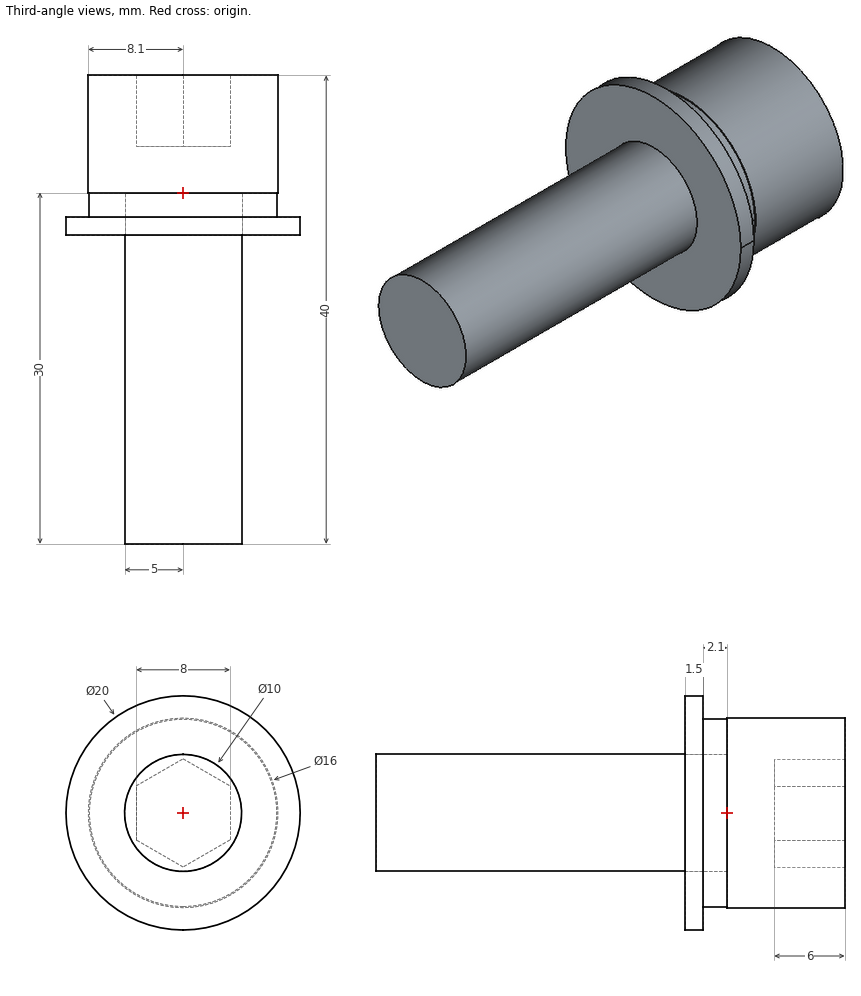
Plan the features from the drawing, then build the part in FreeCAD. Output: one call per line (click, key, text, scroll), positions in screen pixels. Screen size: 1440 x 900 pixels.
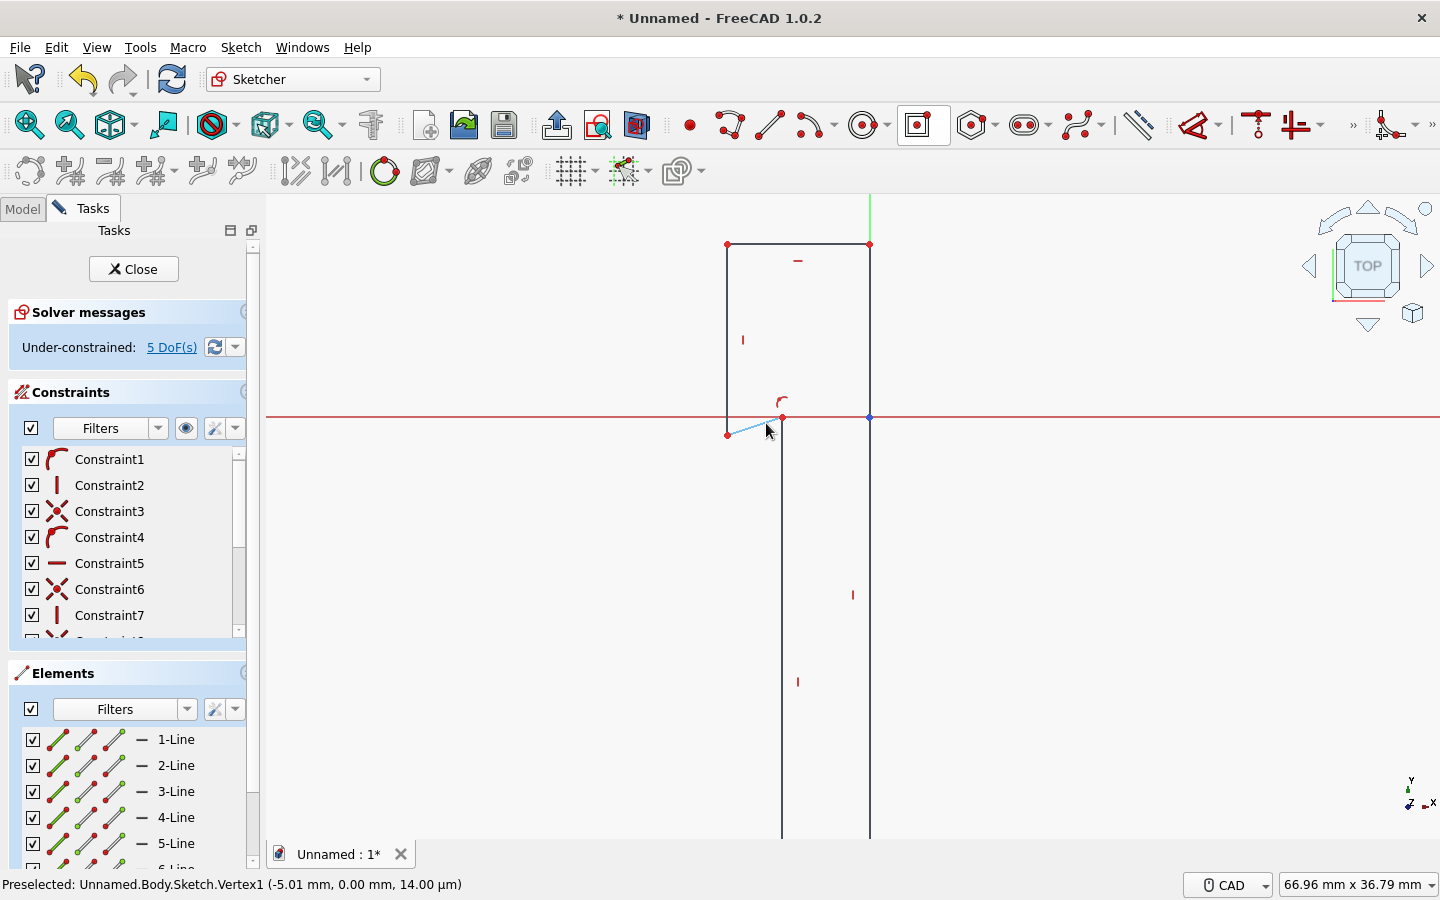
click(766, 423)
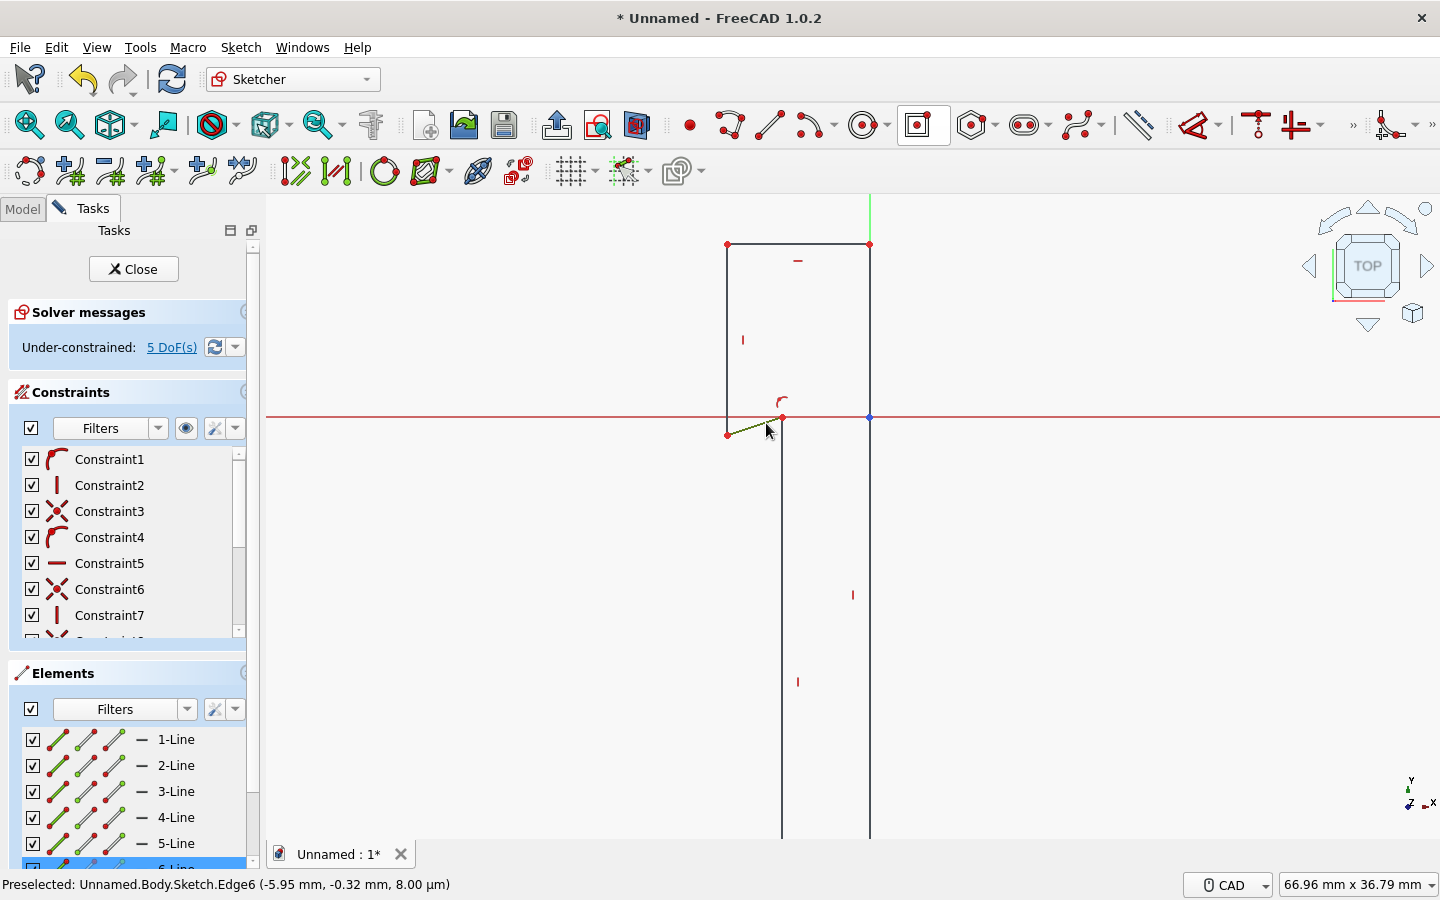
key(h)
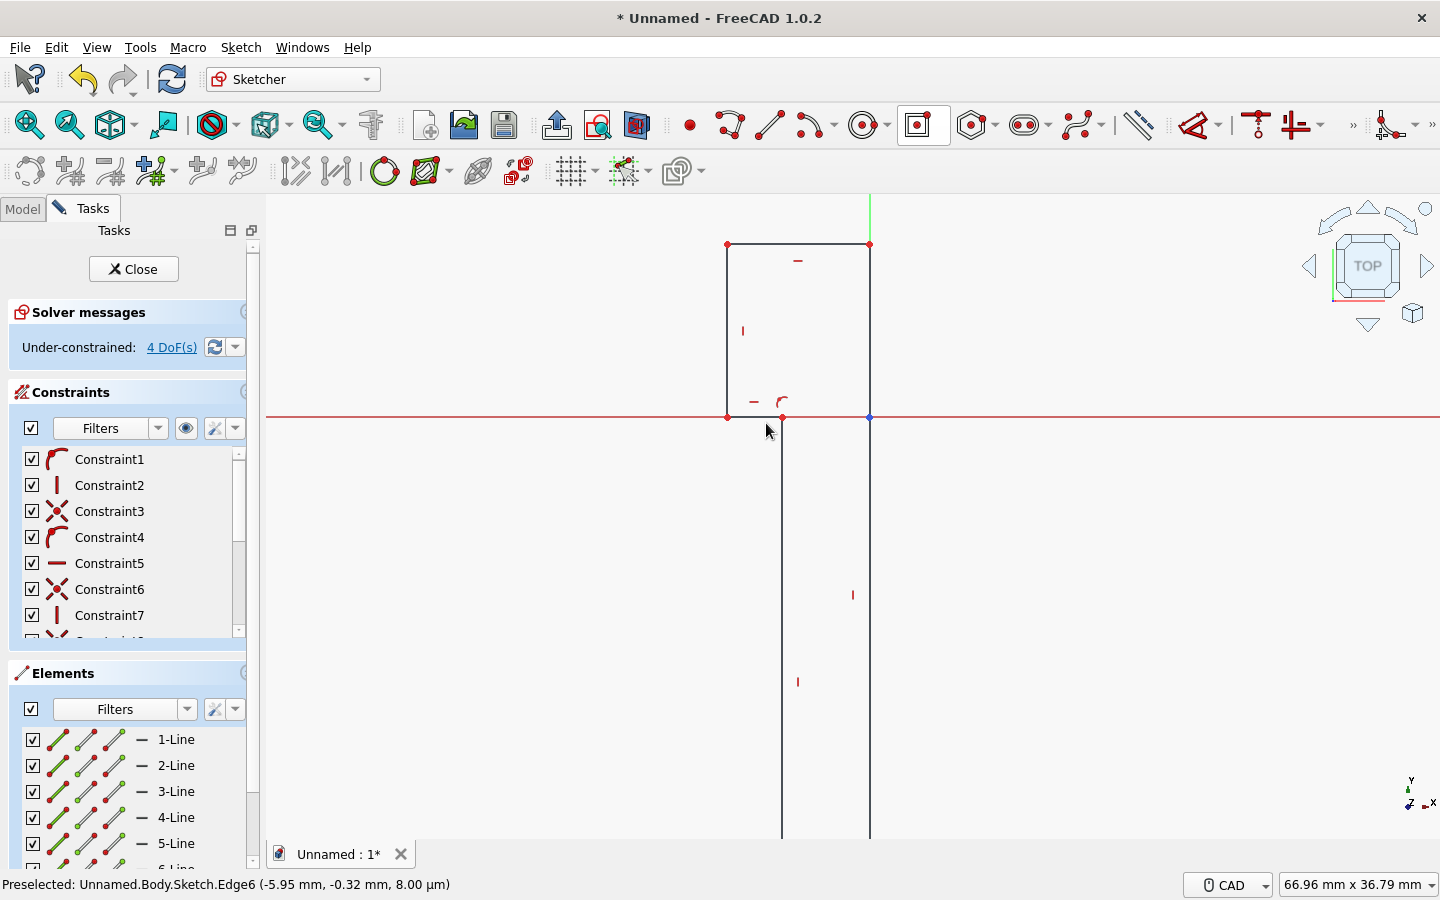
key(d)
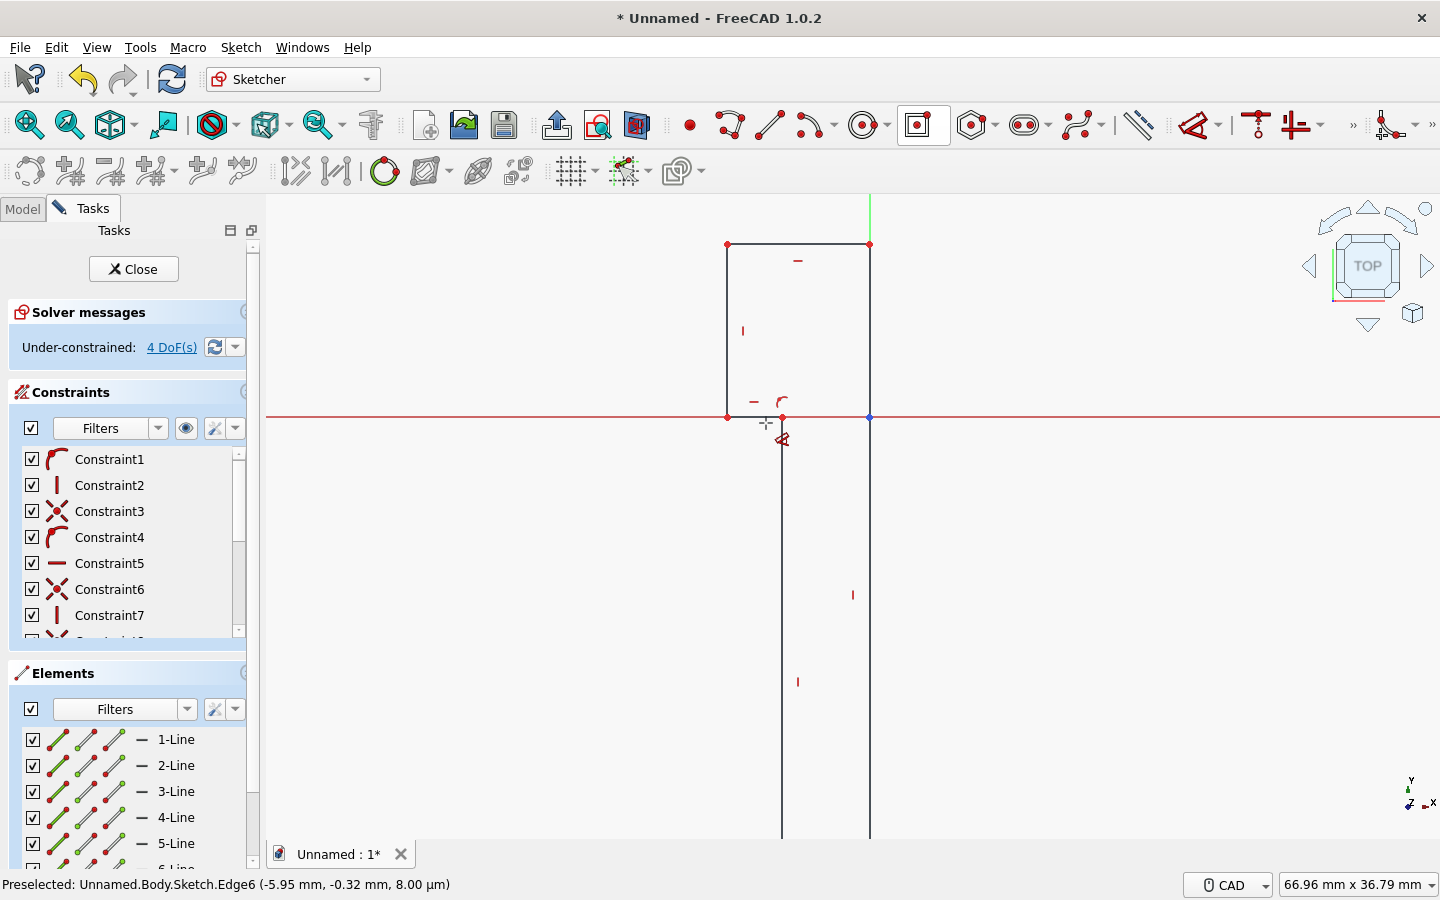
scroll(767, 424, down, 3)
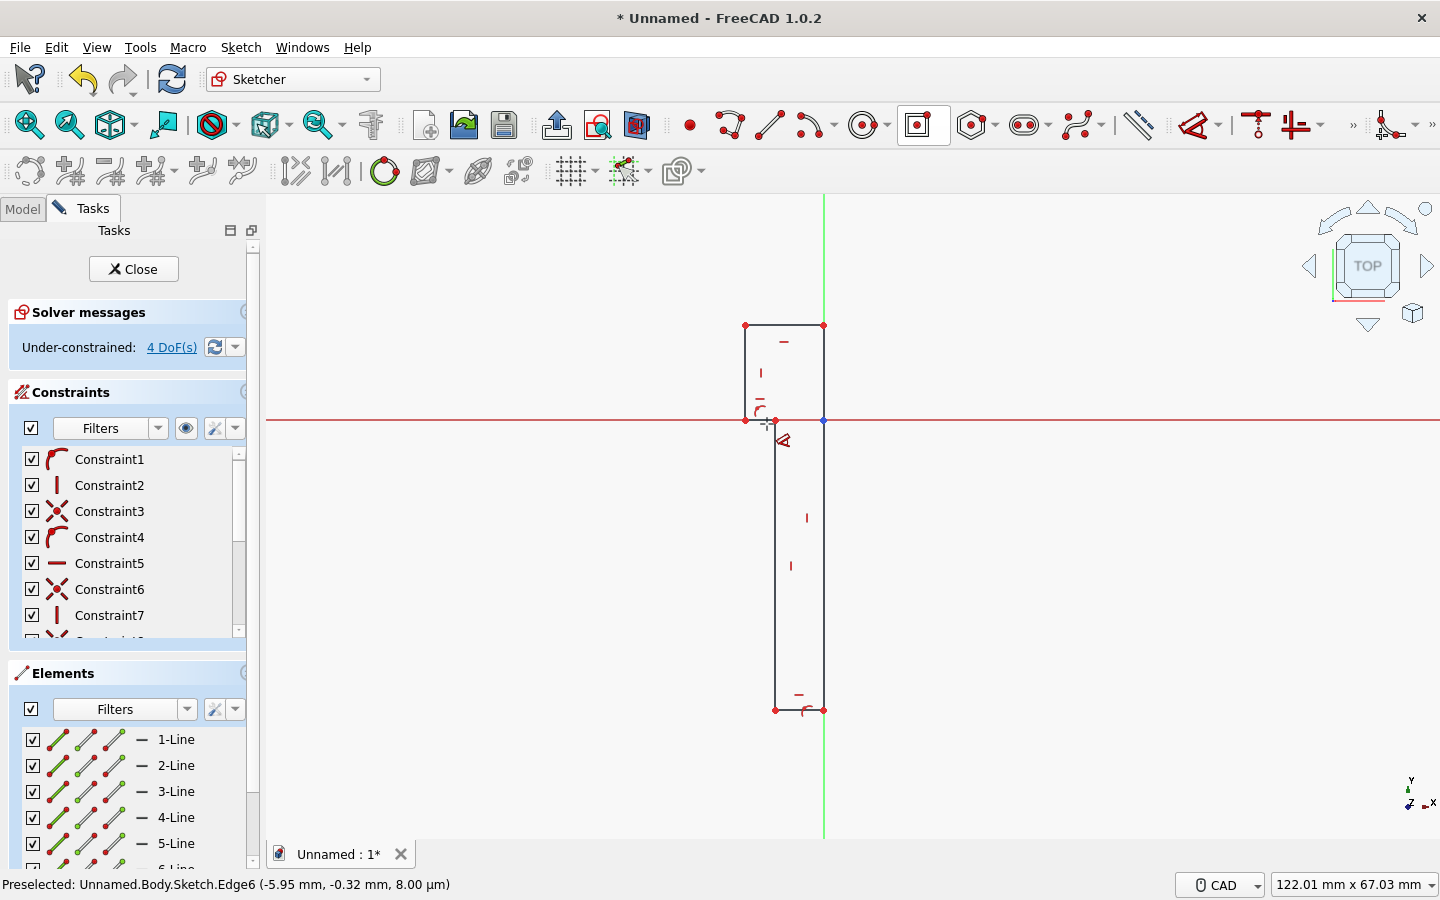
click(790, 710)
click(800, 744)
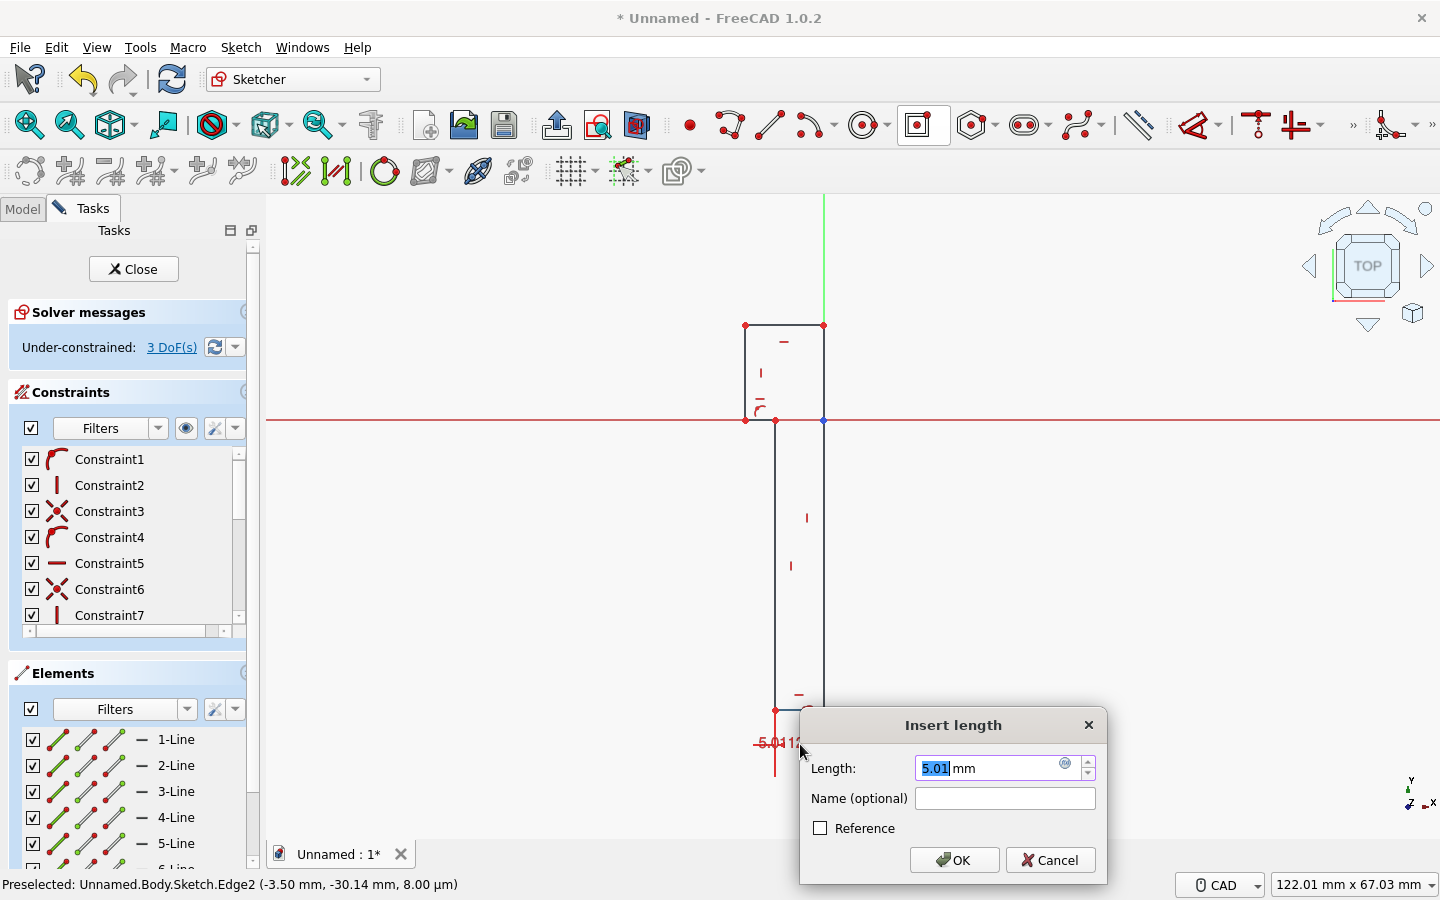
text(5)
key(Return)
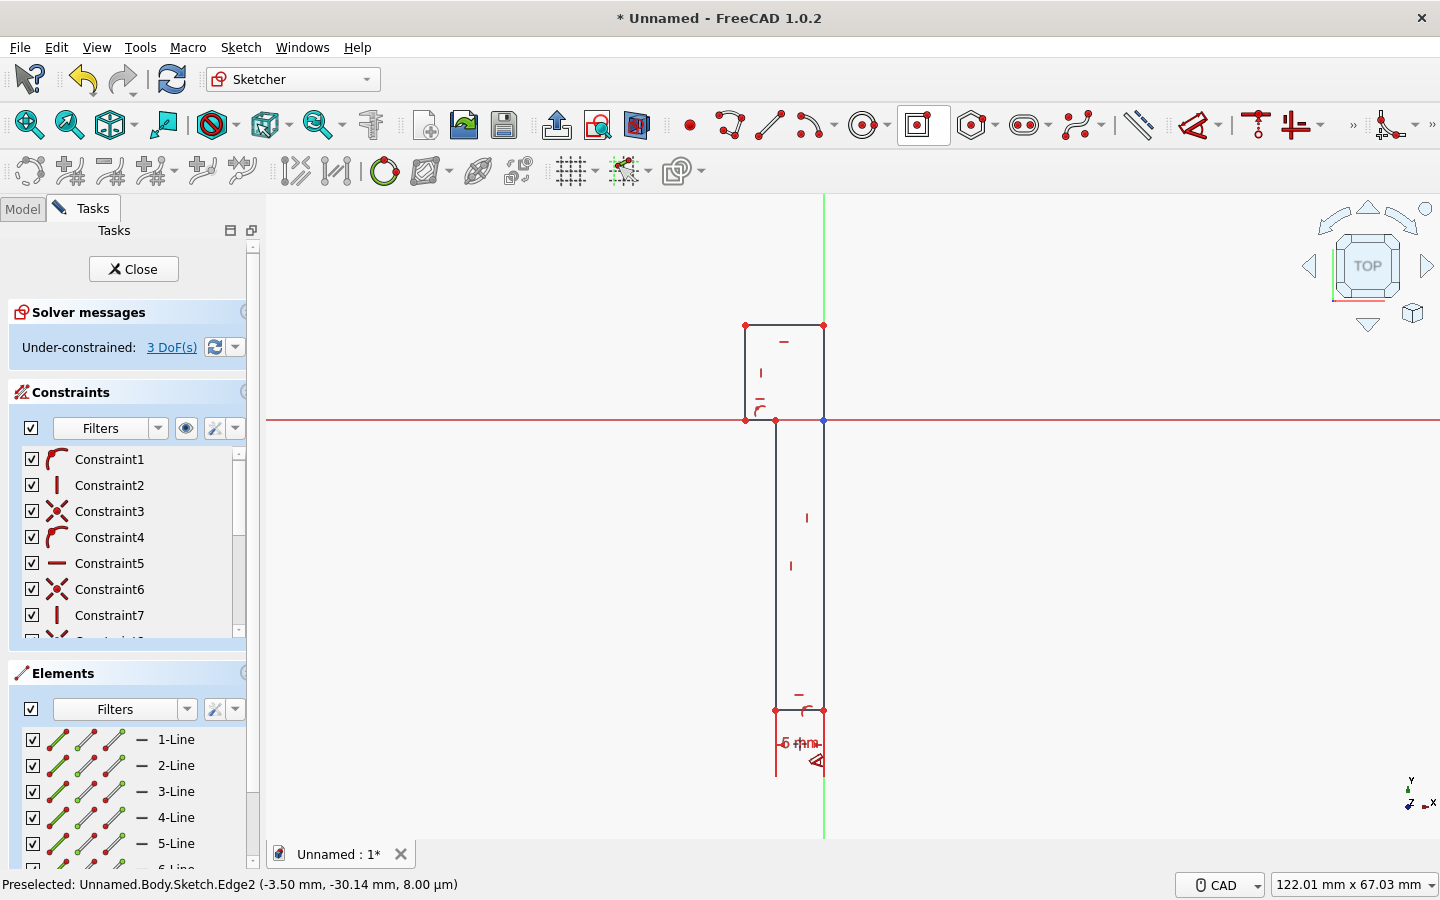
click(776, 507)
click(742, 565)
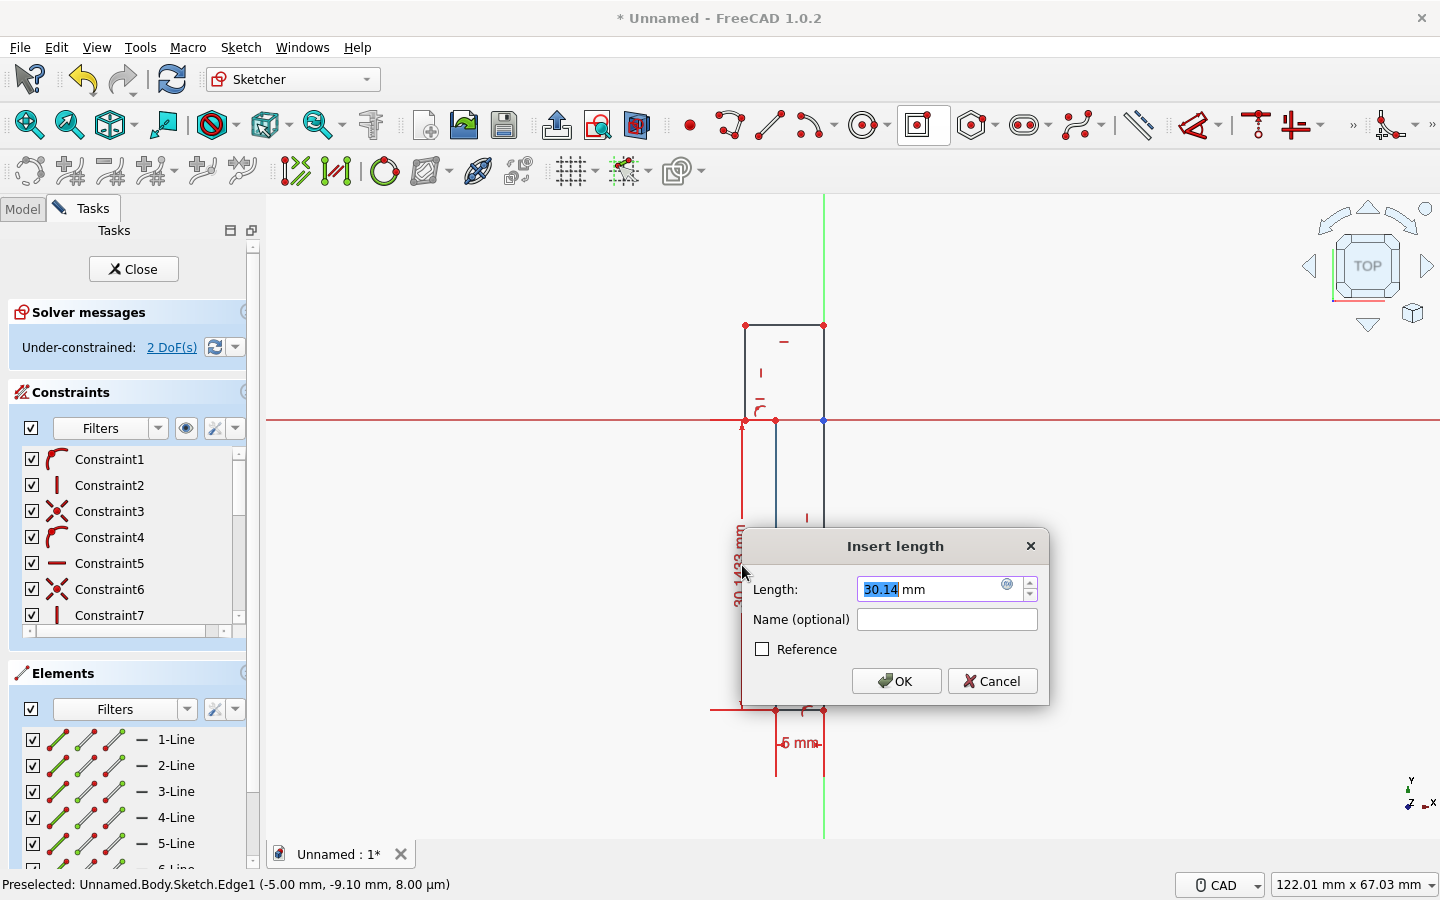
text(30)
key(Return)